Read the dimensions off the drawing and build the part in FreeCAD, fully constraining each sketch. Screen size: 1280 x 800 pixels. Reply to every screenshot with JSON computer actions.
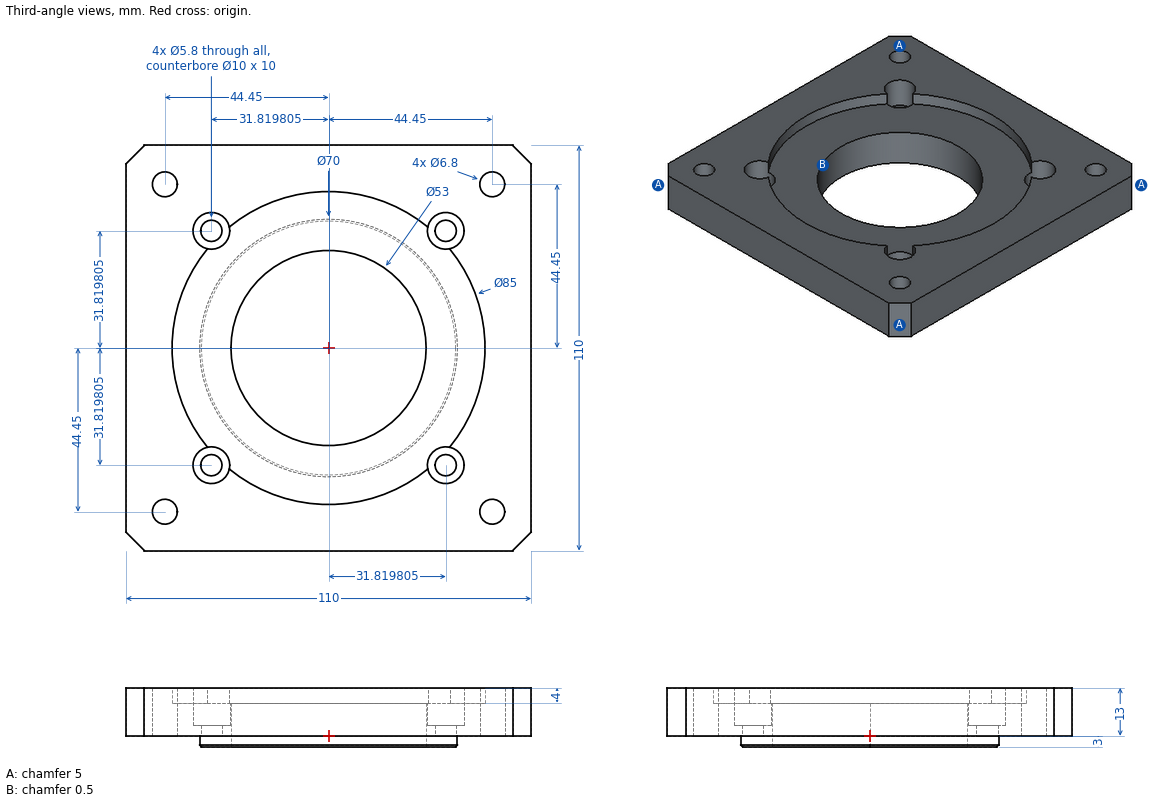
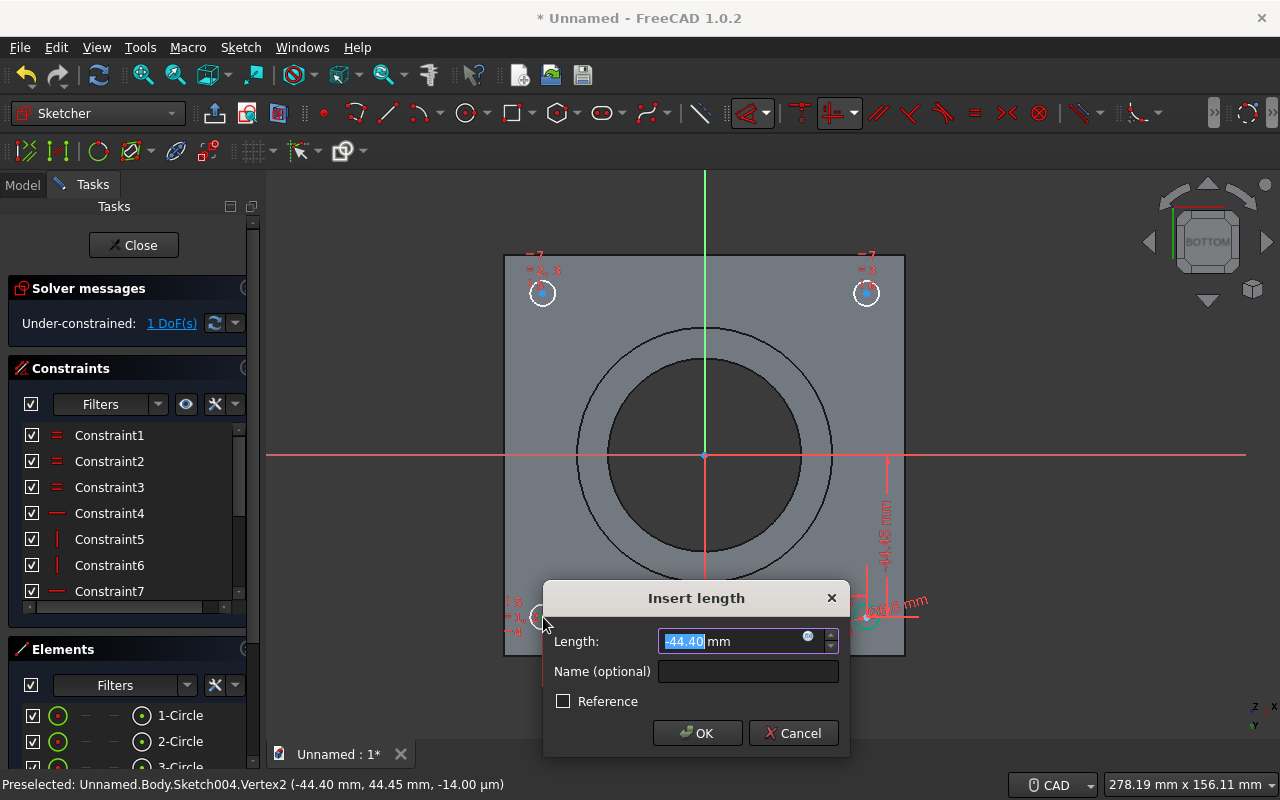
{"action": "type", "text": "-44.45"}
{"action": "key", "text": "Return"}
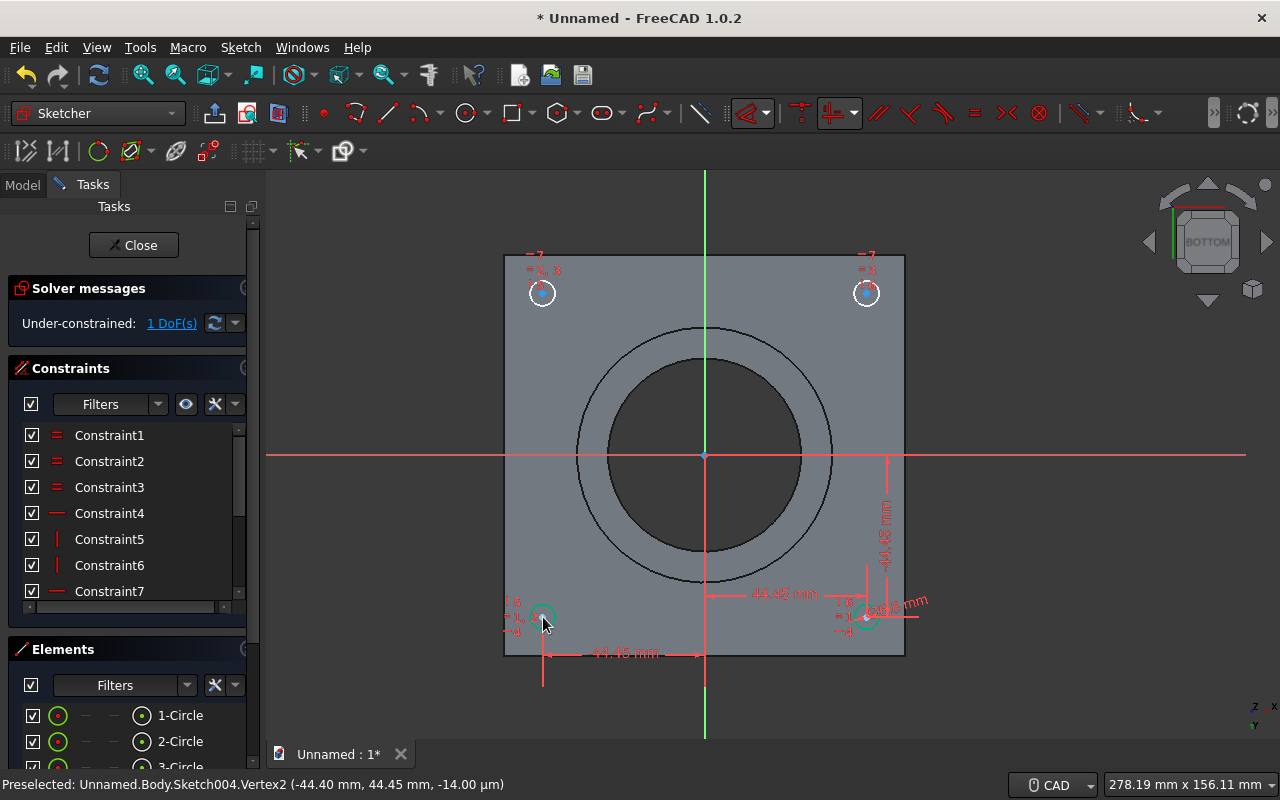
{"action": "left_click", "coordinate": [543, 293]}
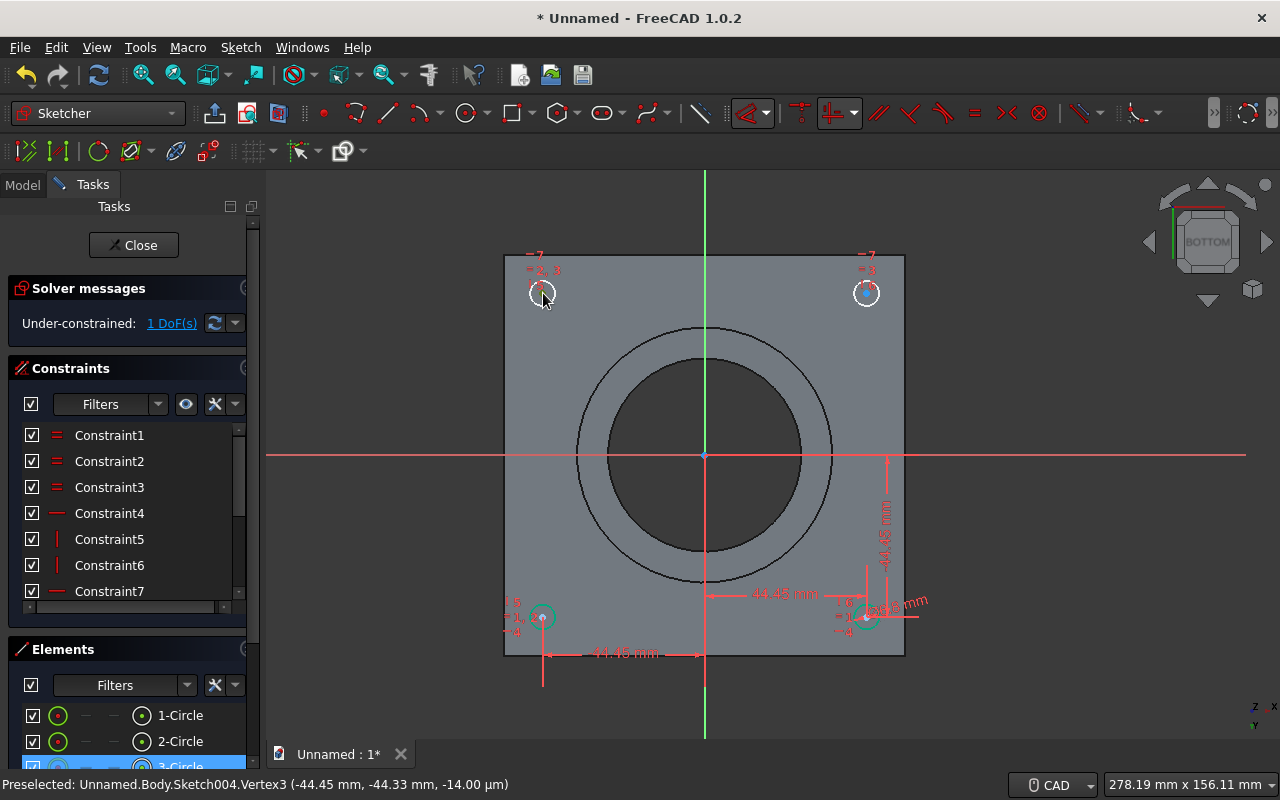
{"action": "left_click", "coordinate": [768, 114]}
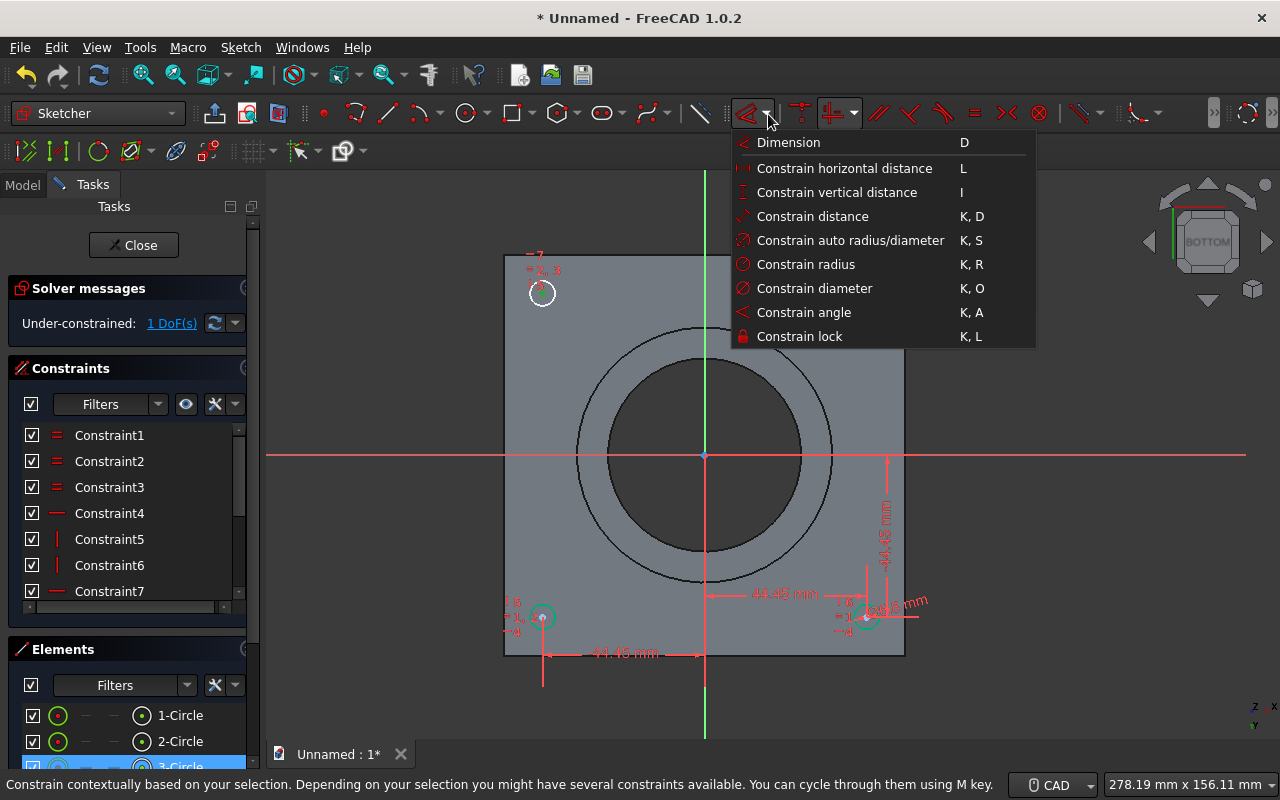
{"action": "left_click", "coordinate": [884, 192]}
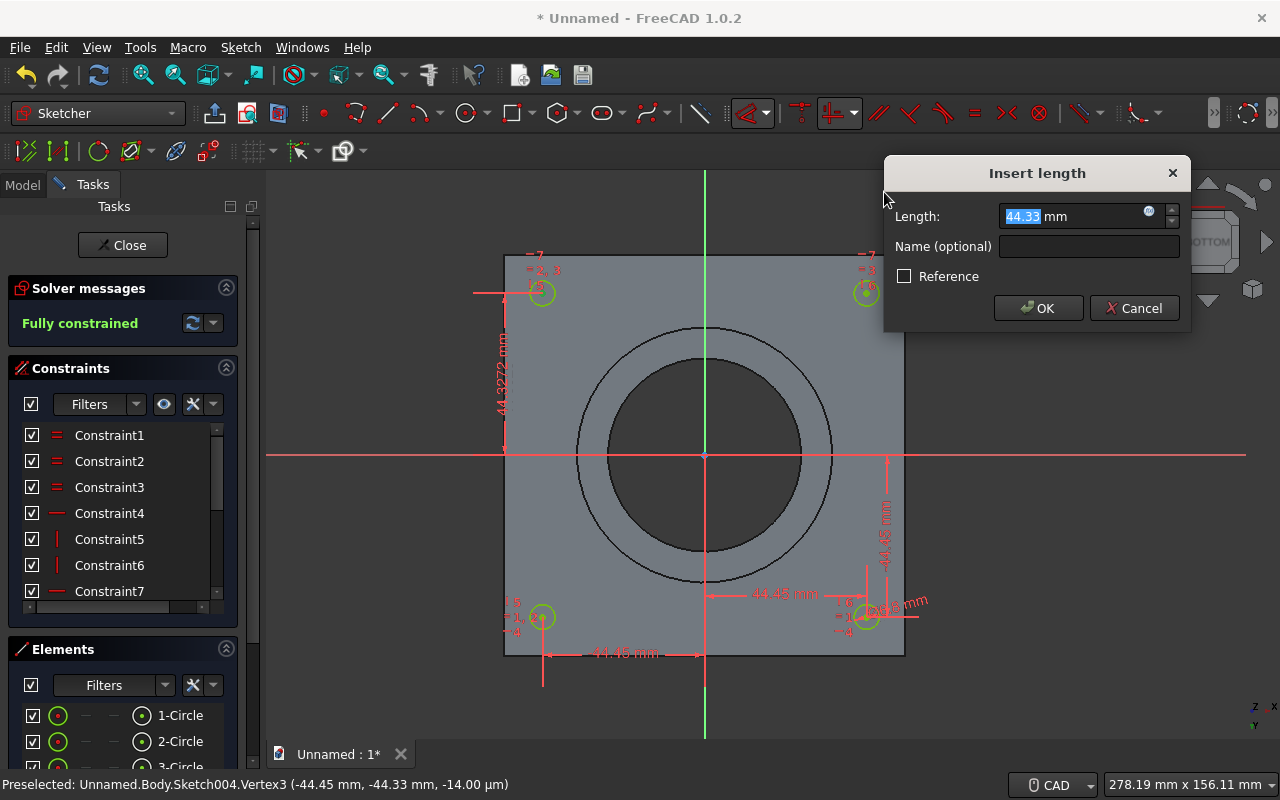
{"action": "type", "text": "44.45"}
{"action": "key", "text": "Return"}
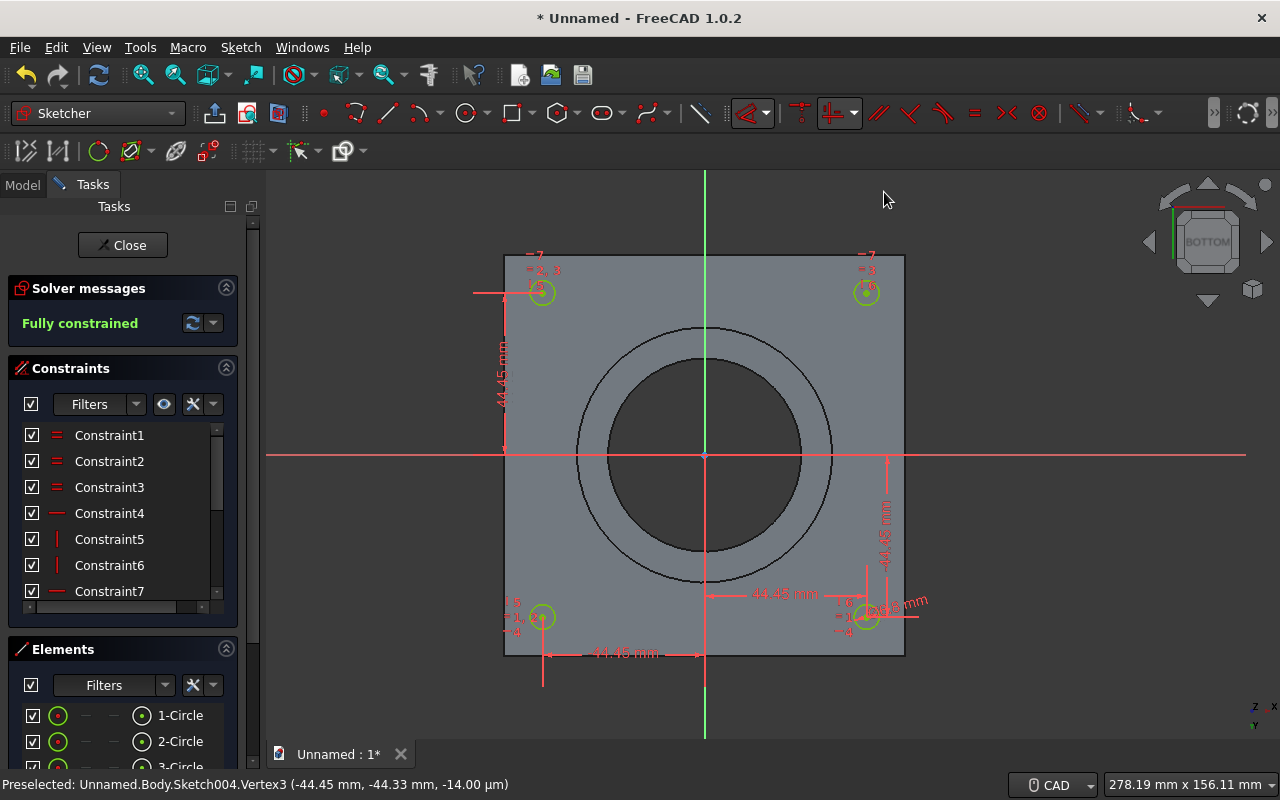
{"action": "left_click", "coordinate": [123, 245]}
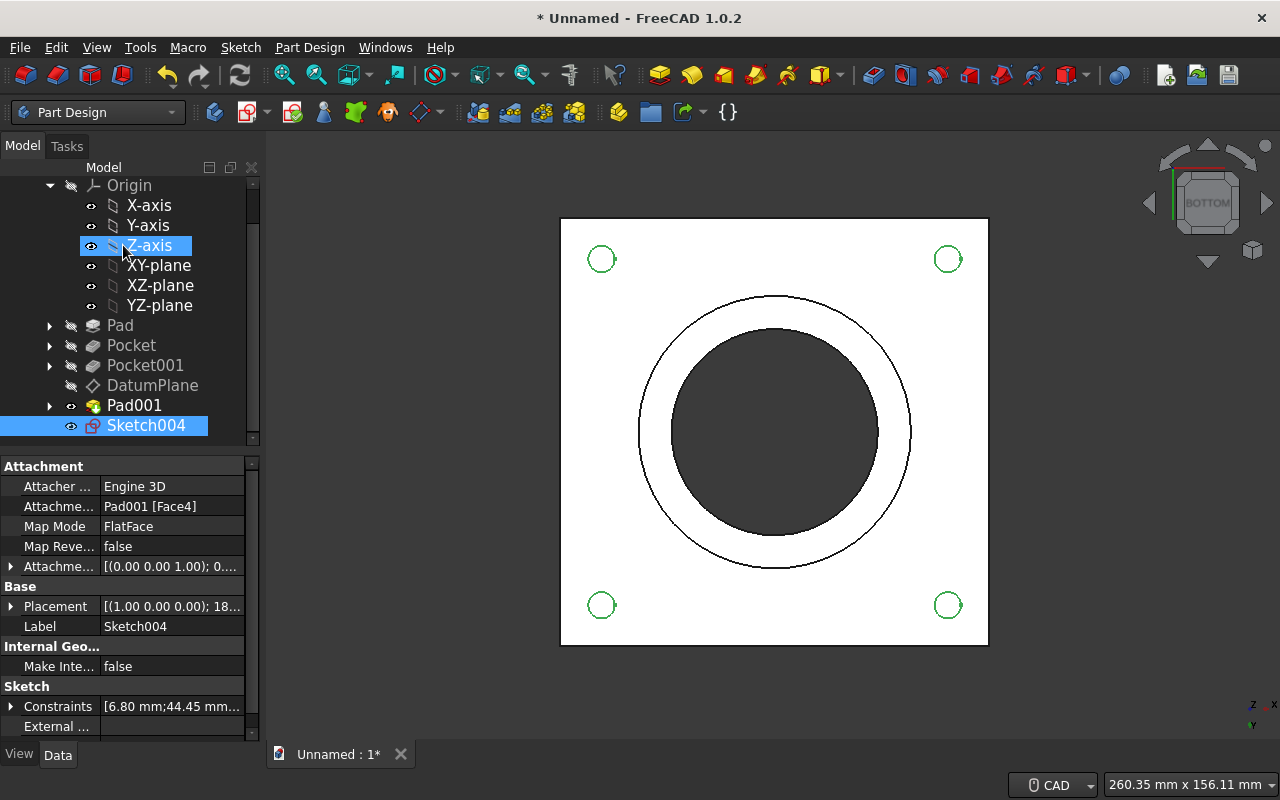
{"action": "left_click", "coordinate": [874, 76]}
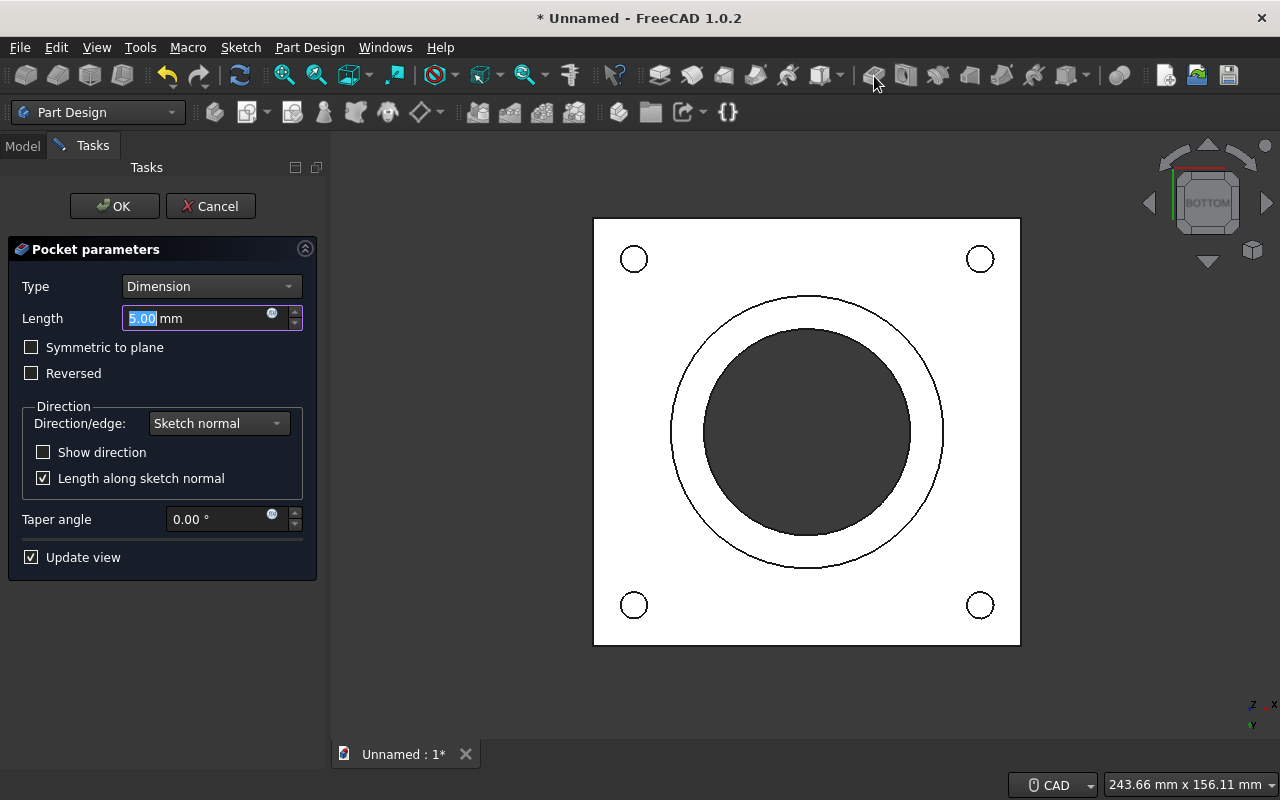
{"action": "left_click", "coordinate": [212, 286]}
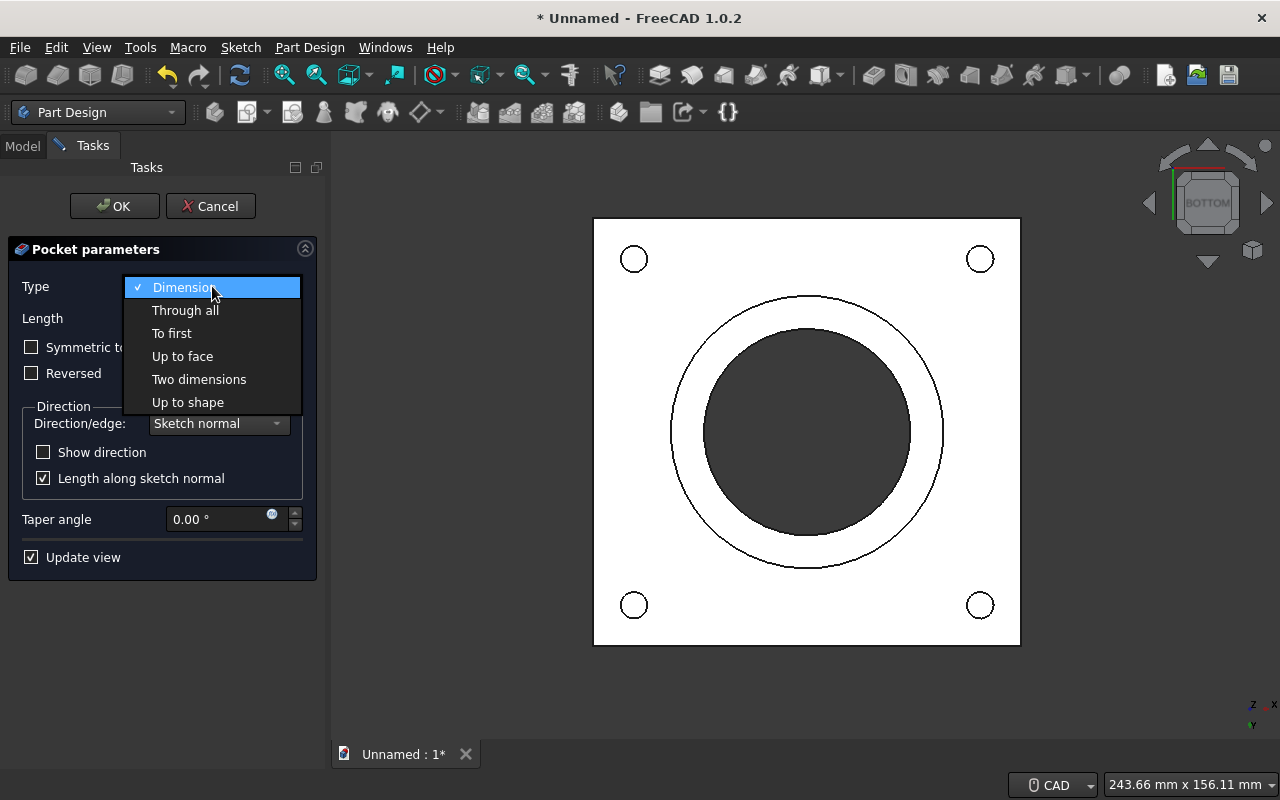
{"action": "left_click", "coordinate": [212, 310]}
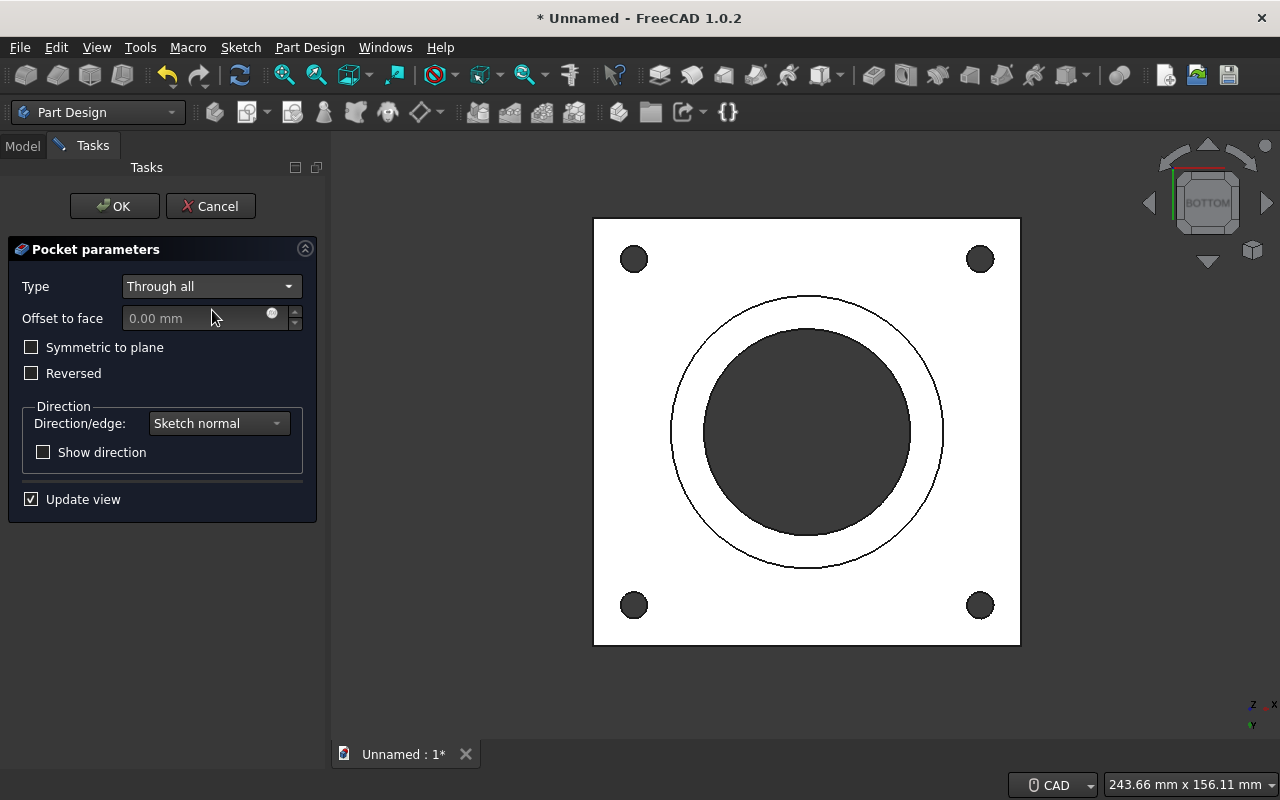
{"action": "left_click", "coordinate": [115, 206]}